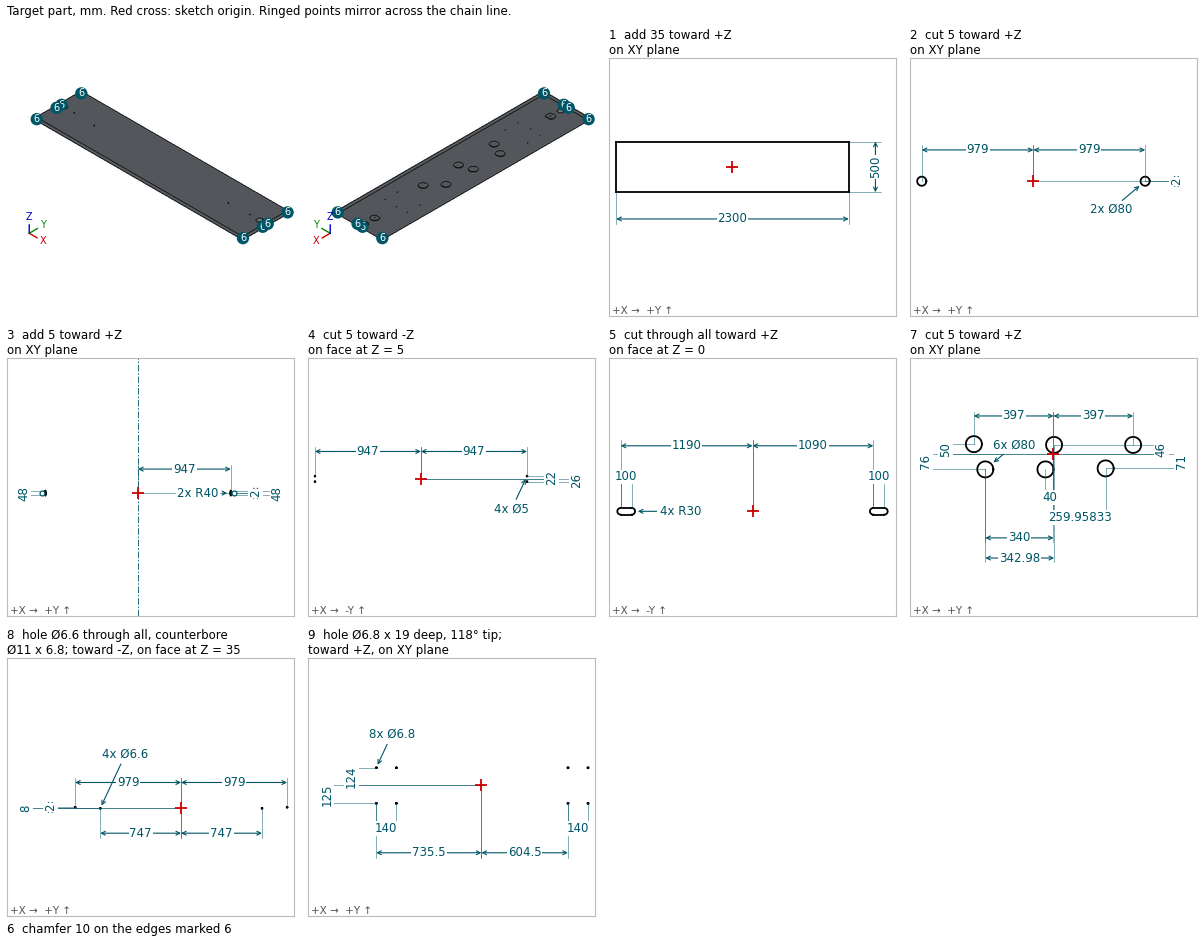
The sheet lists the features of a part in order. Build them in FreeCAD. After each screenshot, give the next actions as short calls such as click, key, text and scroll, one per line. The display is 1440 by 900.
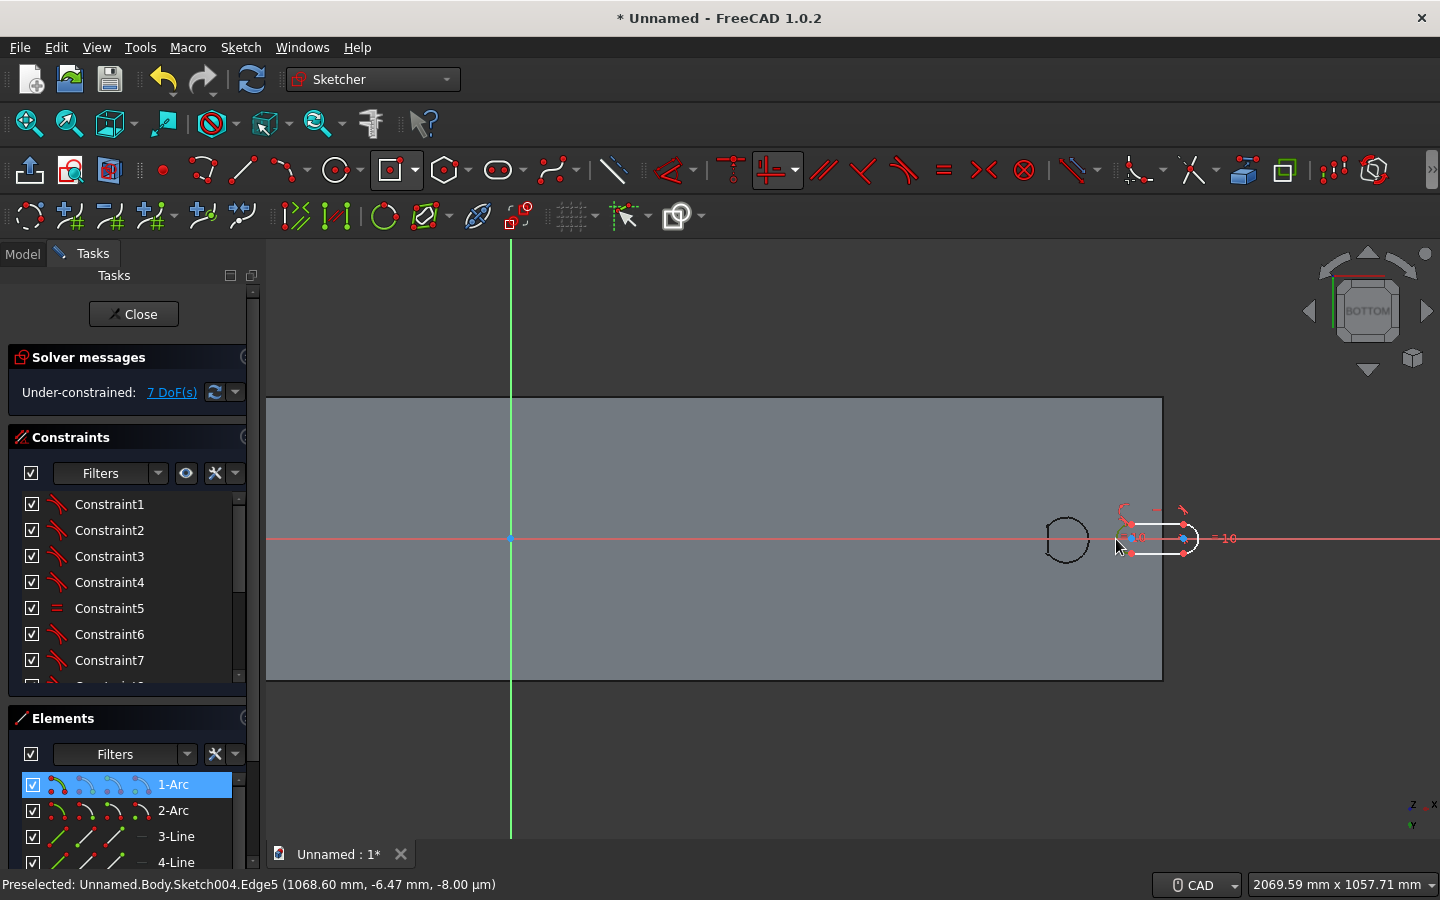
click(944, 170)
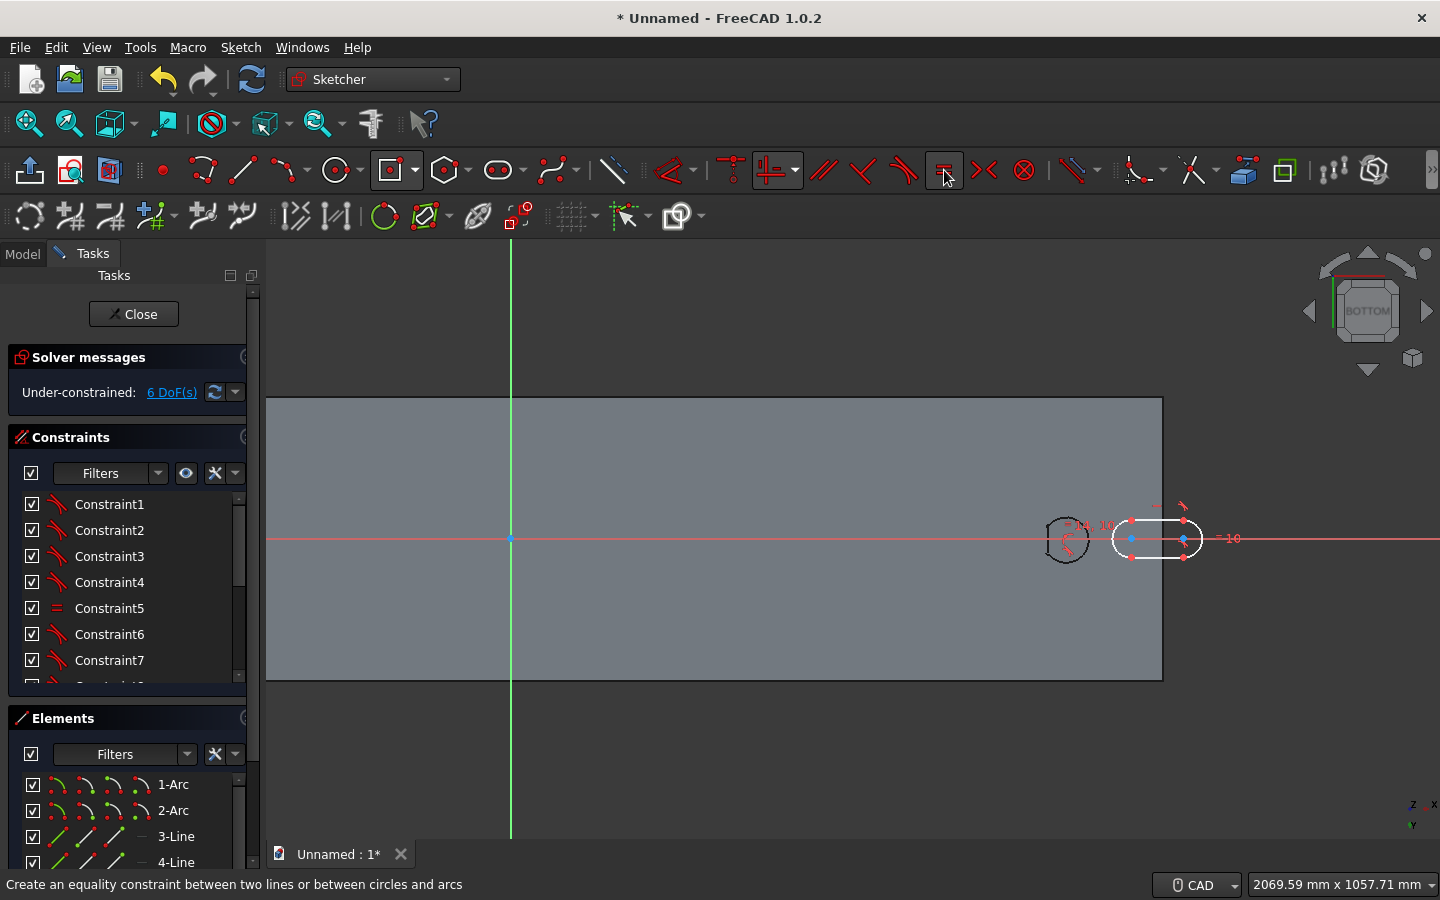
scroll(1117, 539, down, 3)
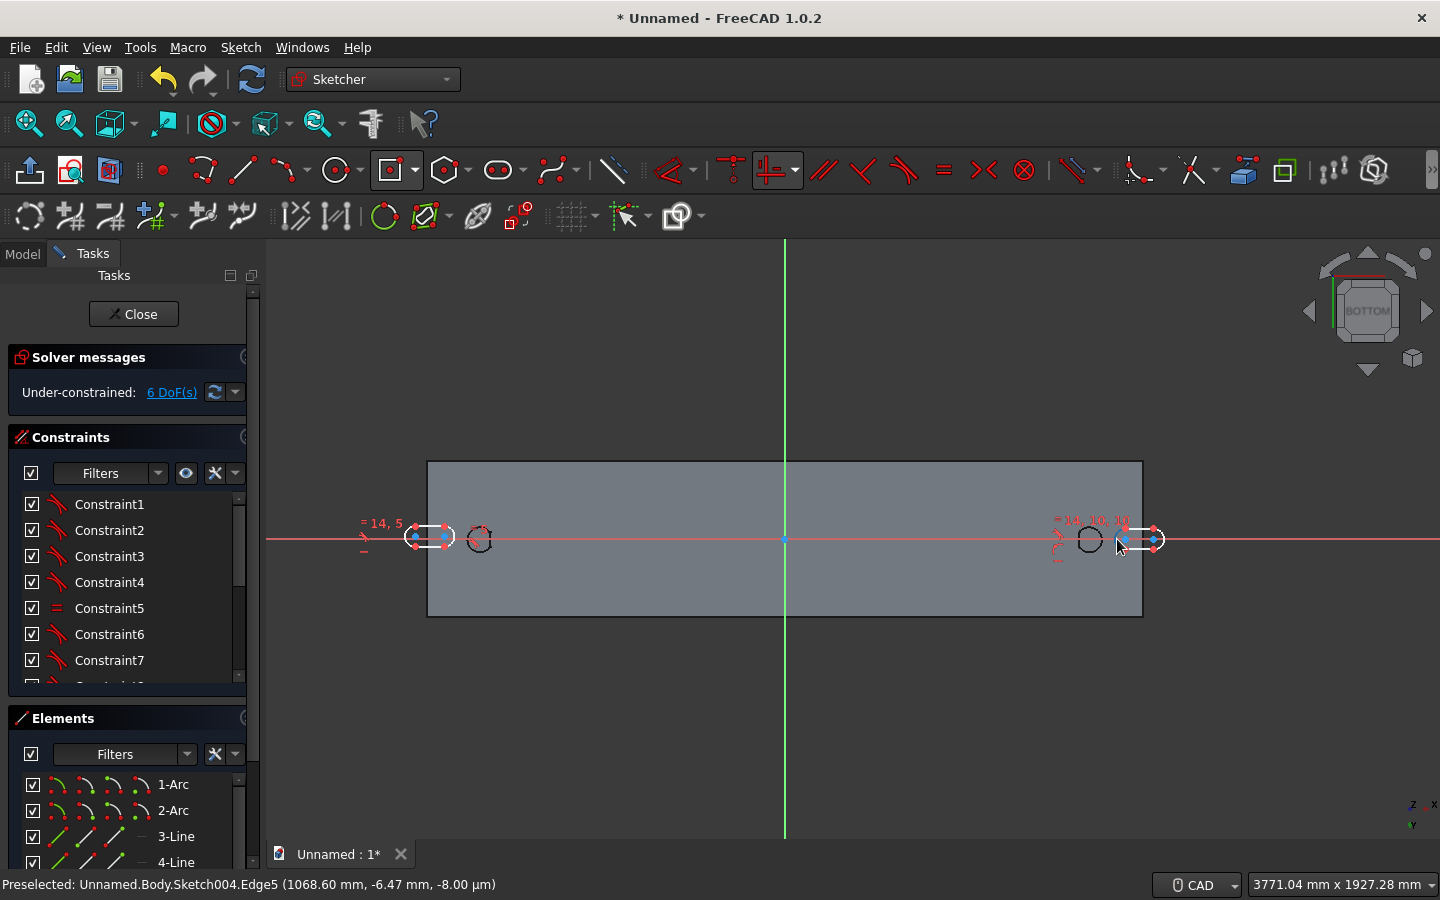
click(415, 536)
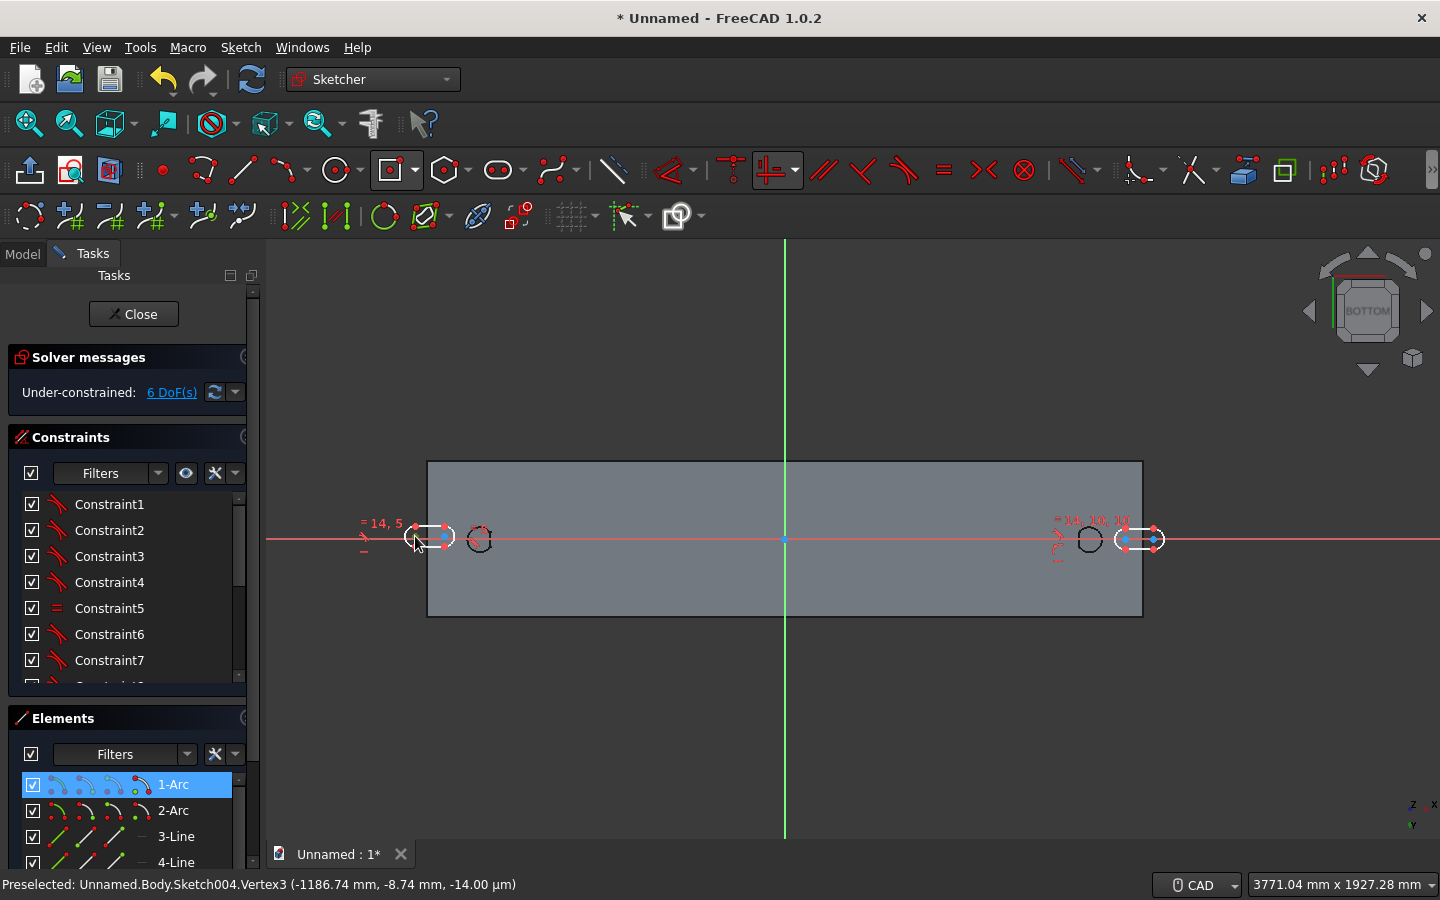
click(504, 539)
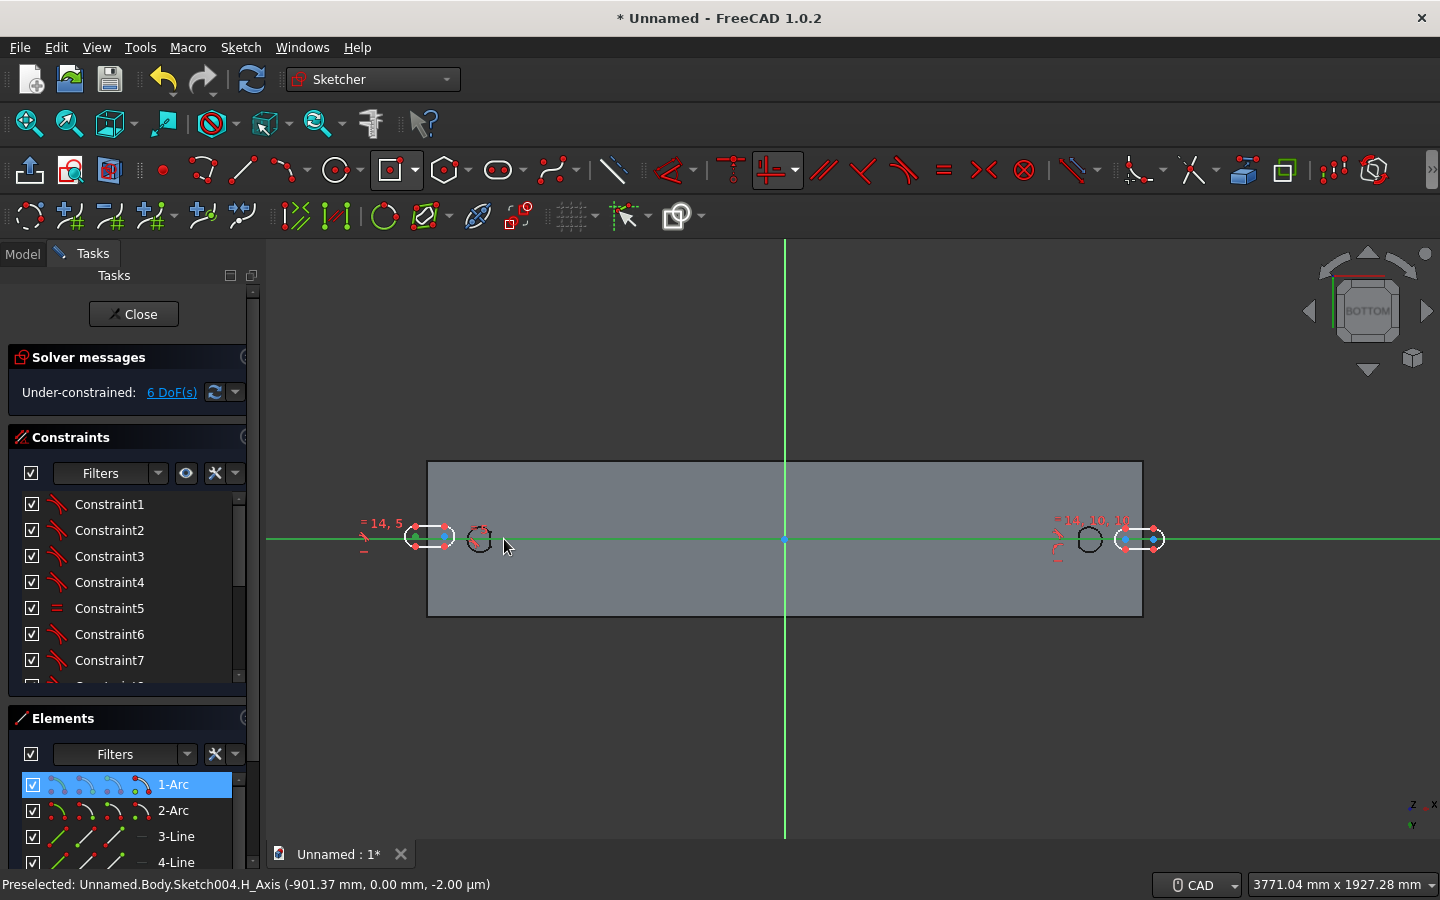
click(732, 170)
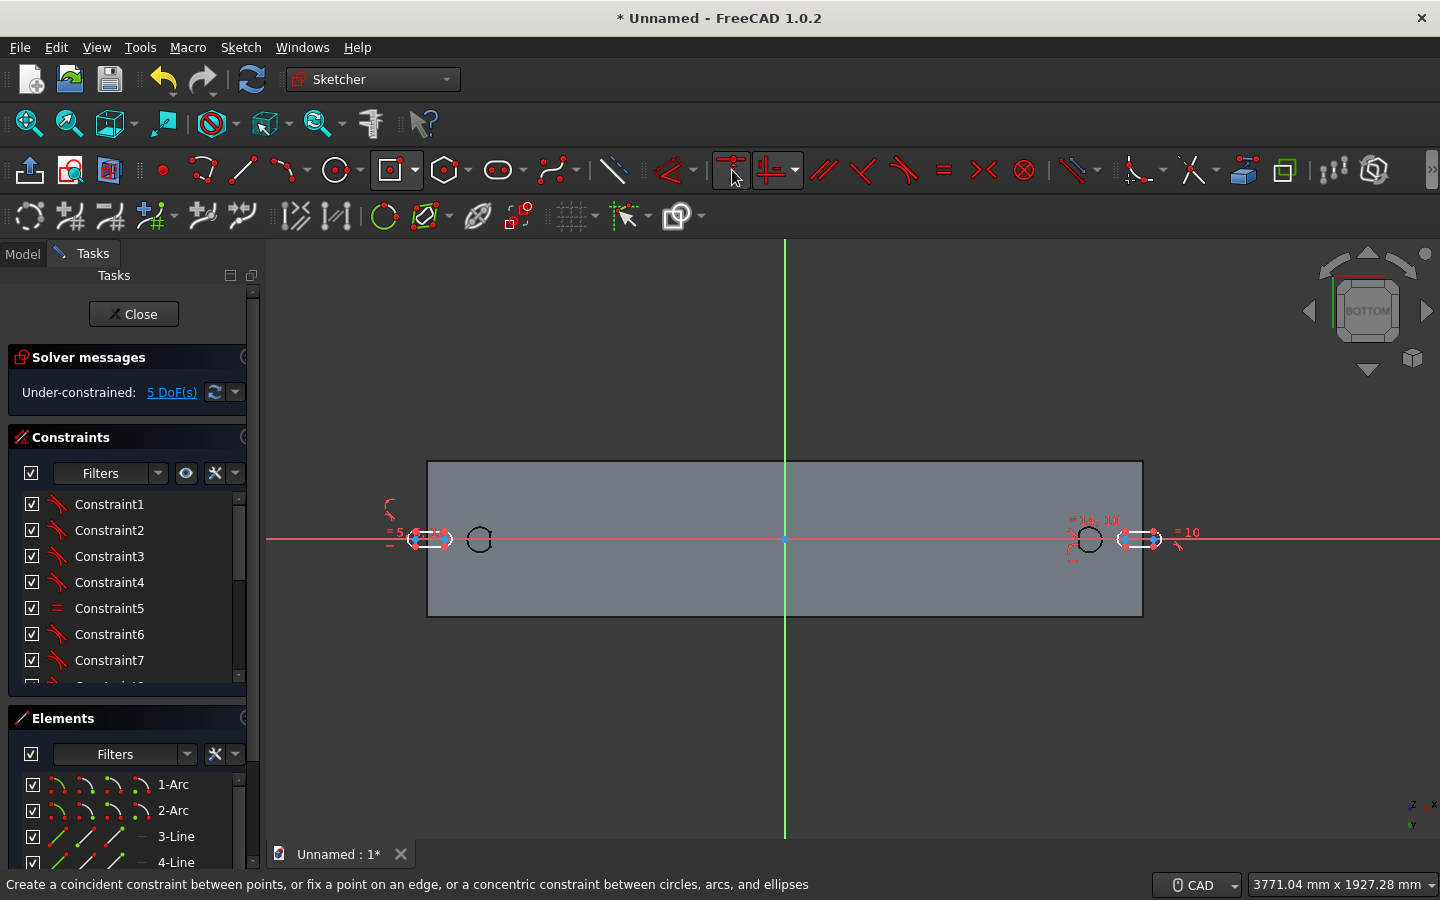
click(668, 170)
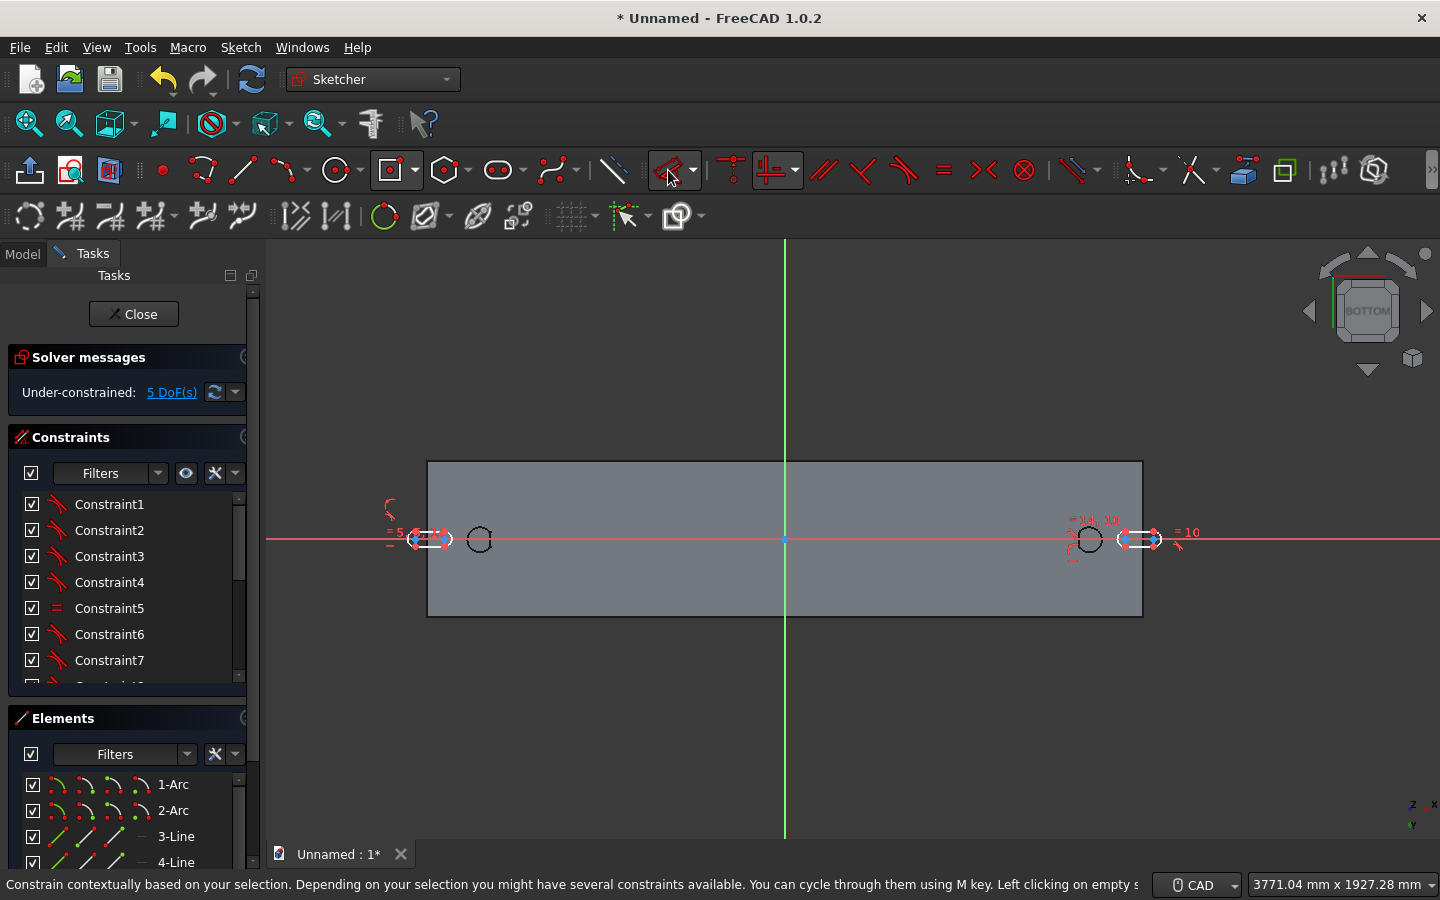
scroll(408, 539, up, 8)